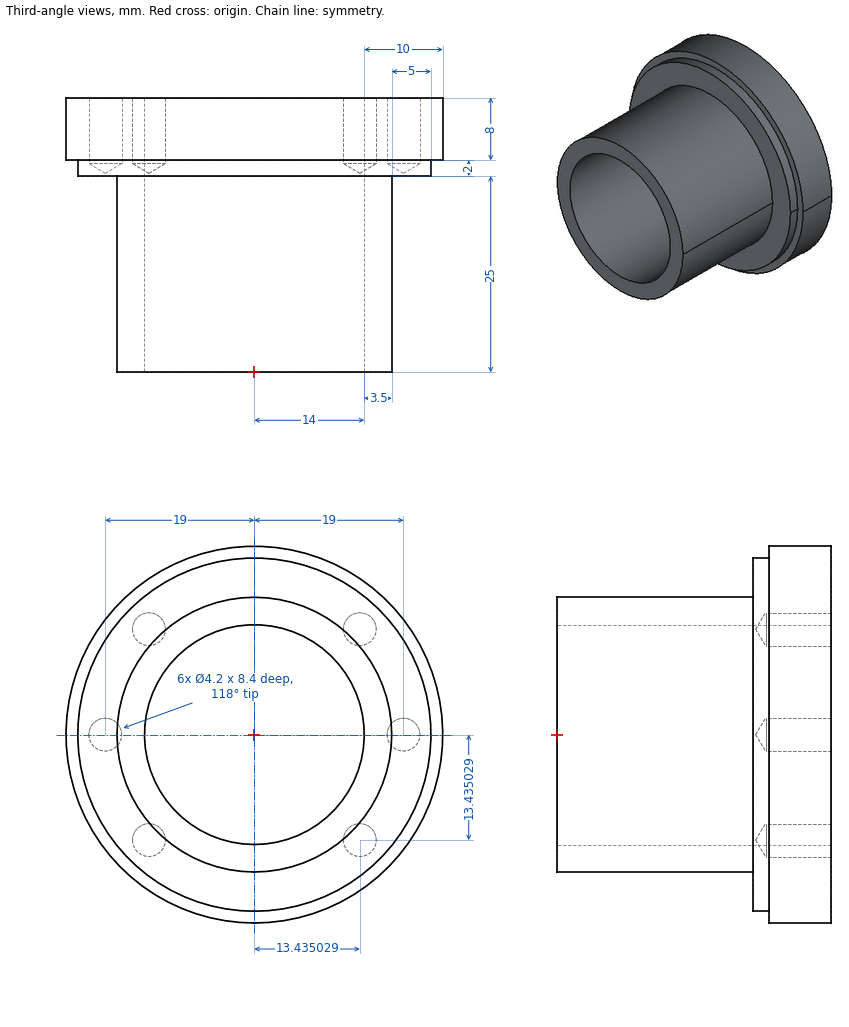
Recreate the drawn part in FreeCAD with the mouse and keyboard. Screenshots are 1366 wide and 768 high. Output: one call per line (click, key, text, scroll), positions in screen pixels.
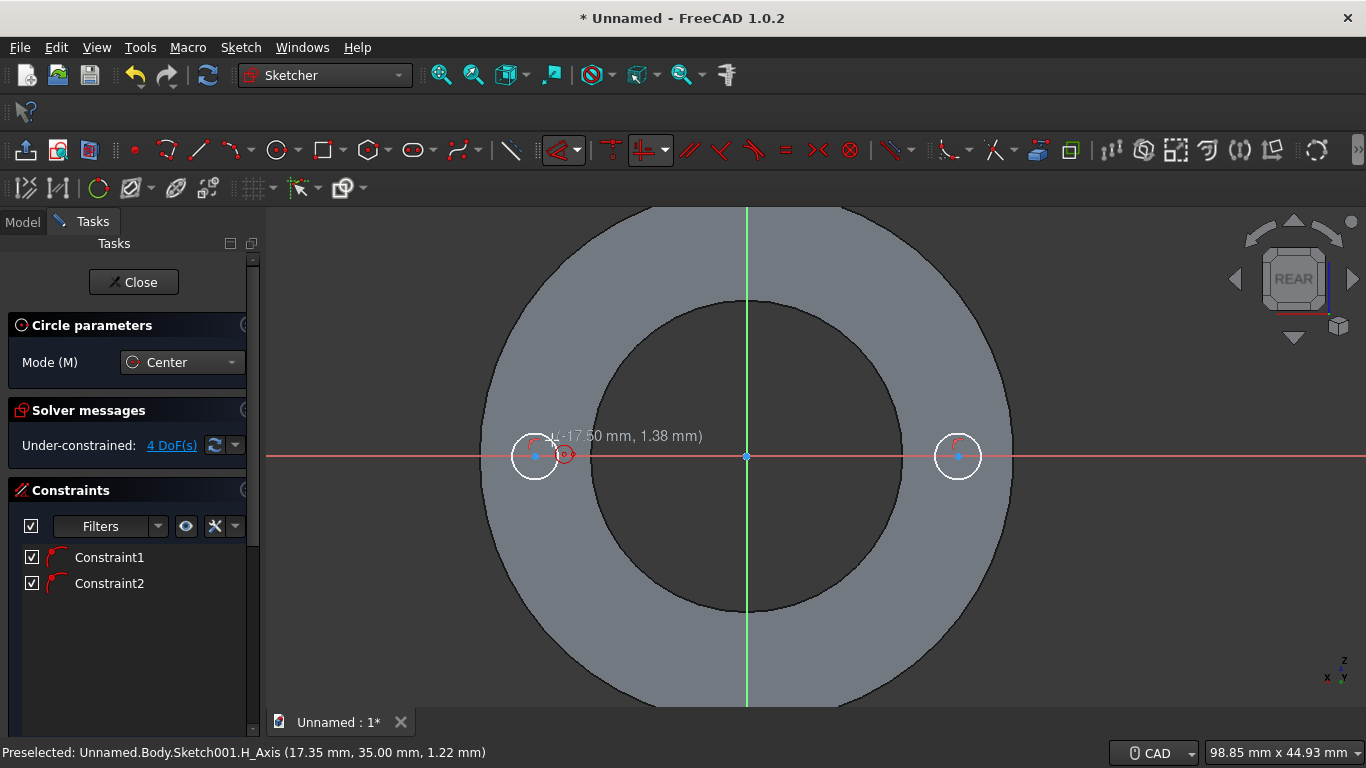
click(597, 606)
click(614, 589)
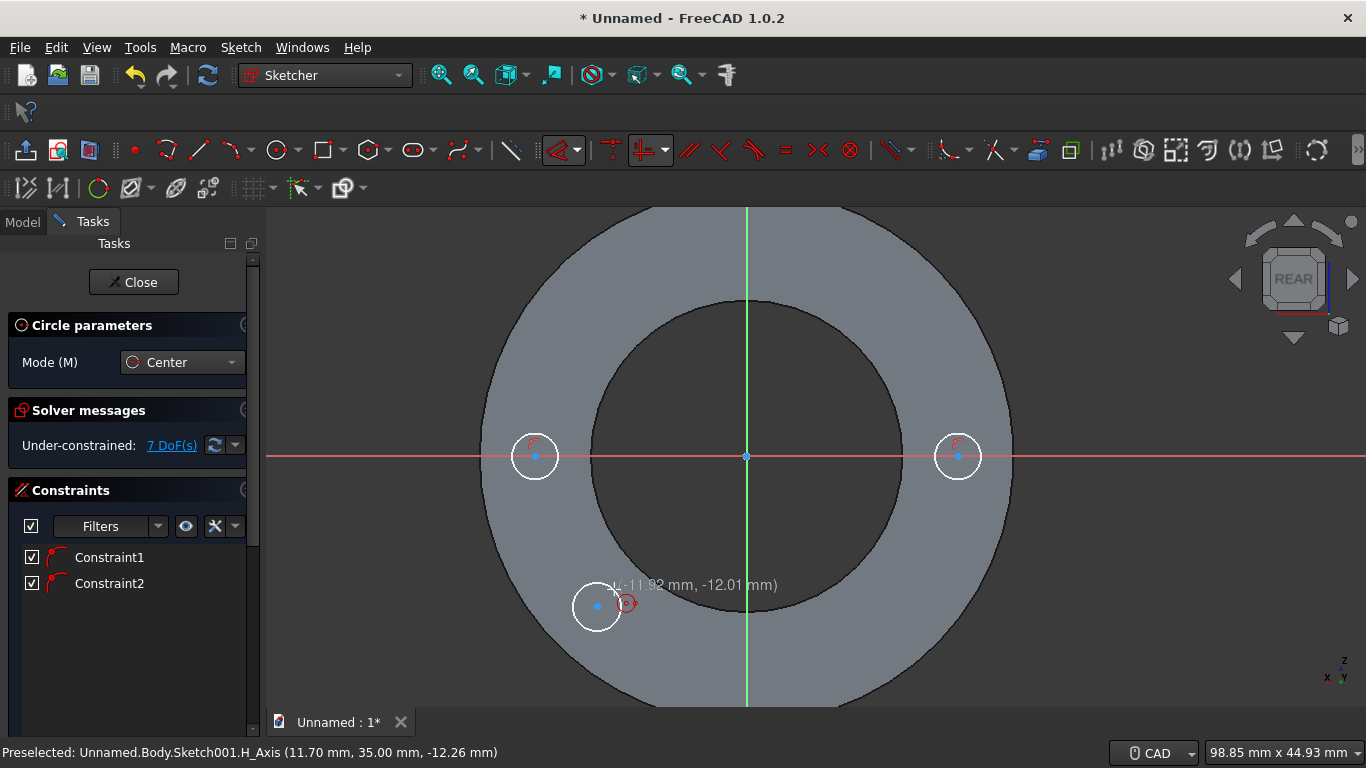
click(597, 307)
click(614, 290)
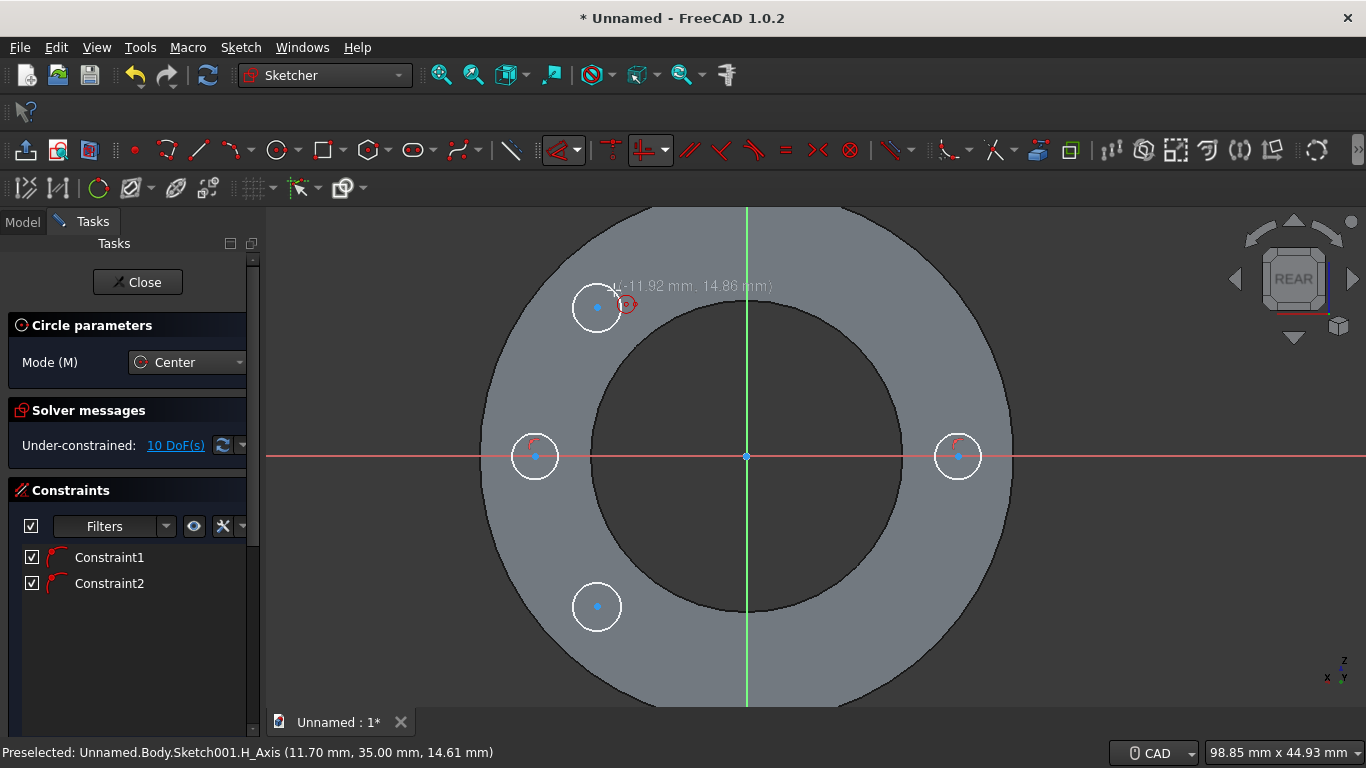
click(896, 307)
click(913, 290)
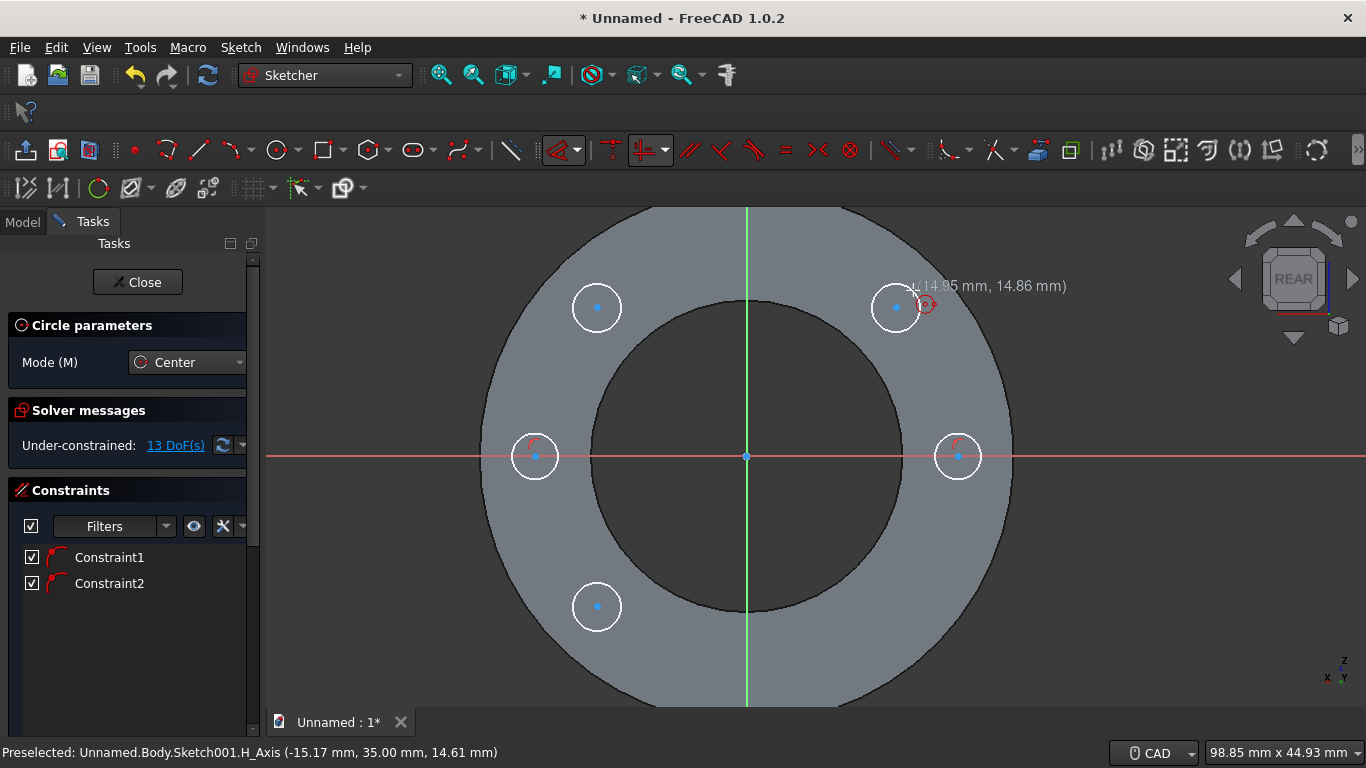
click(896, 606)
click(913, 589)
key(Escape)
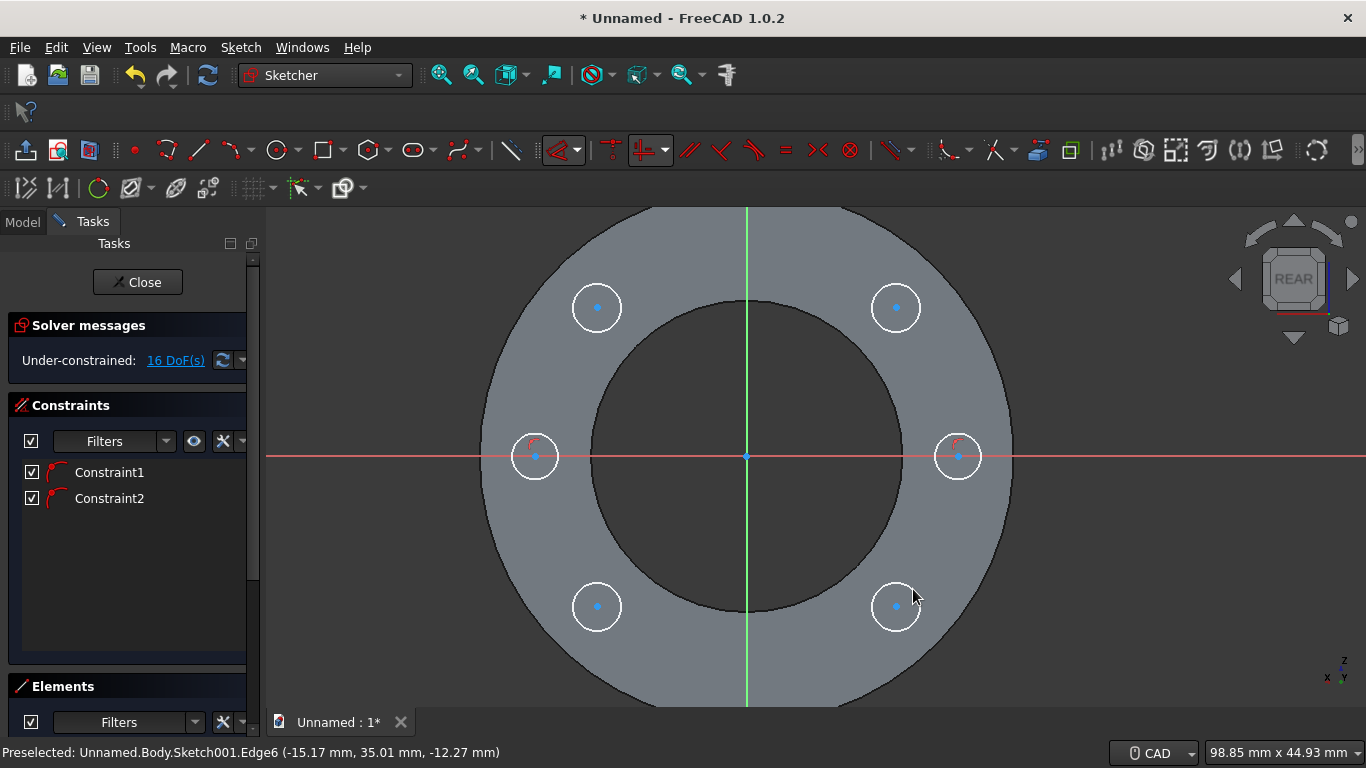
click(974, 440)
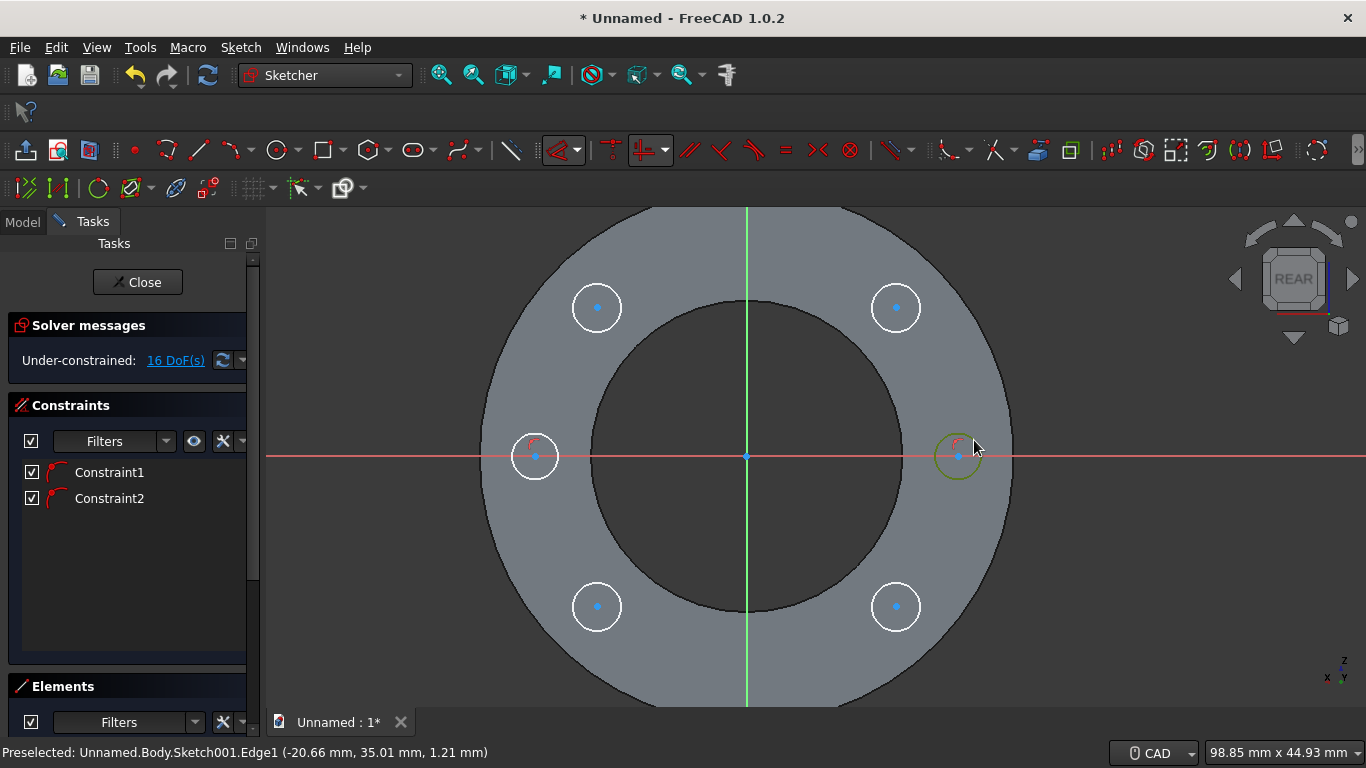
click(551, 440)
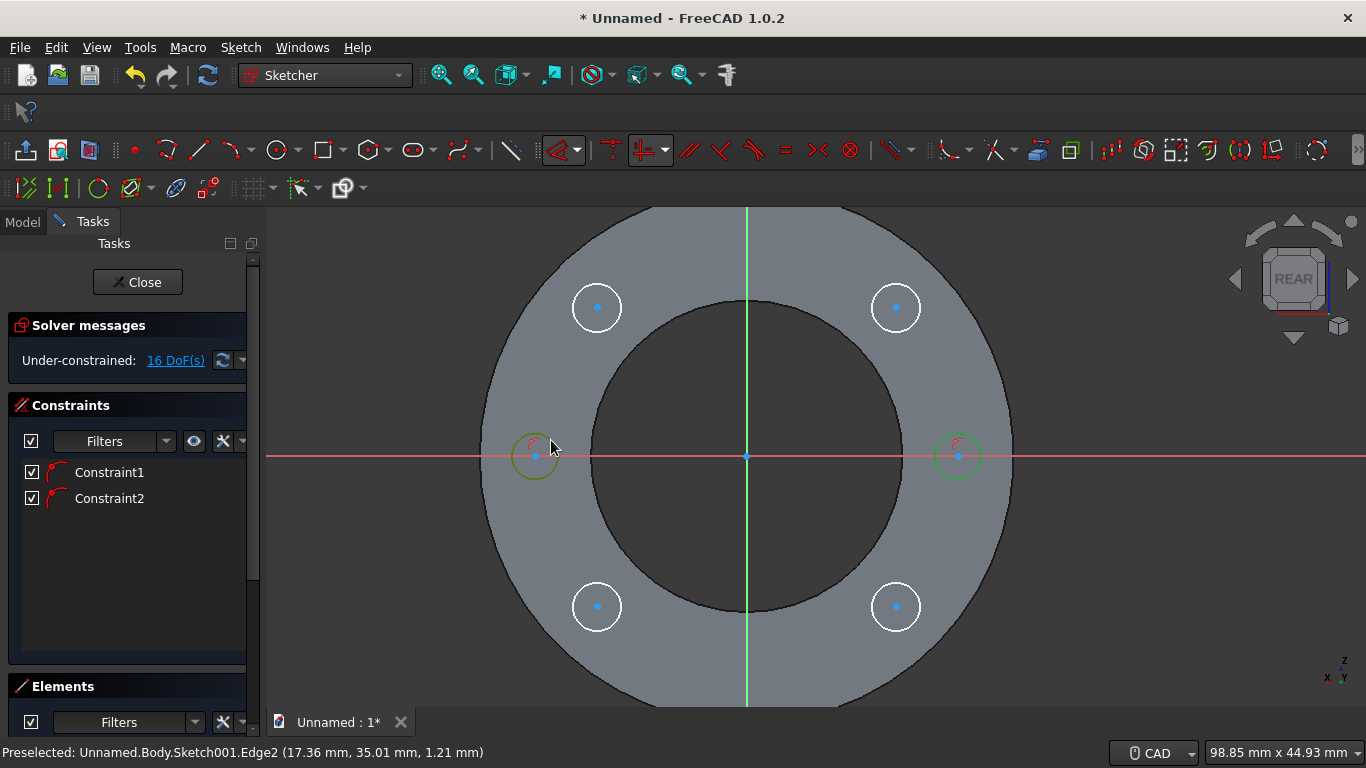
click(614, 590)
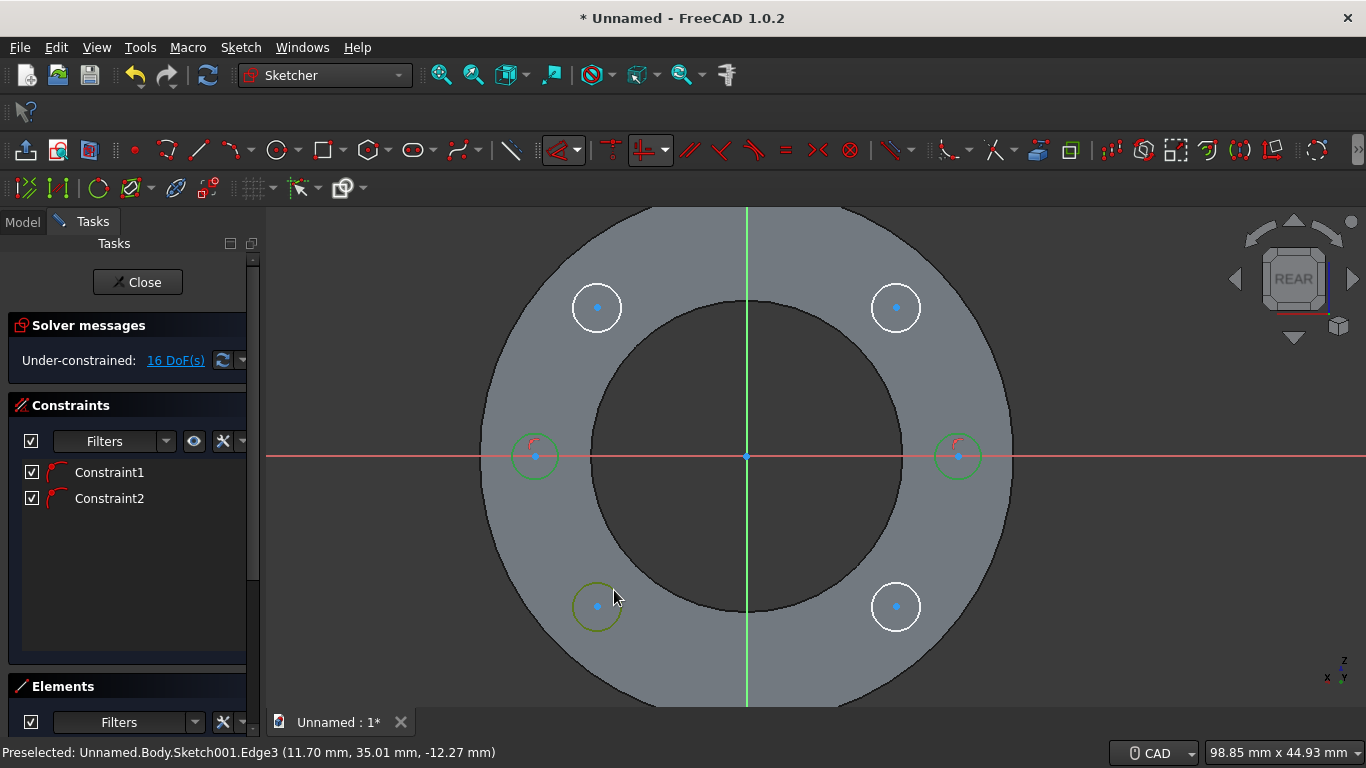
click(614, 291)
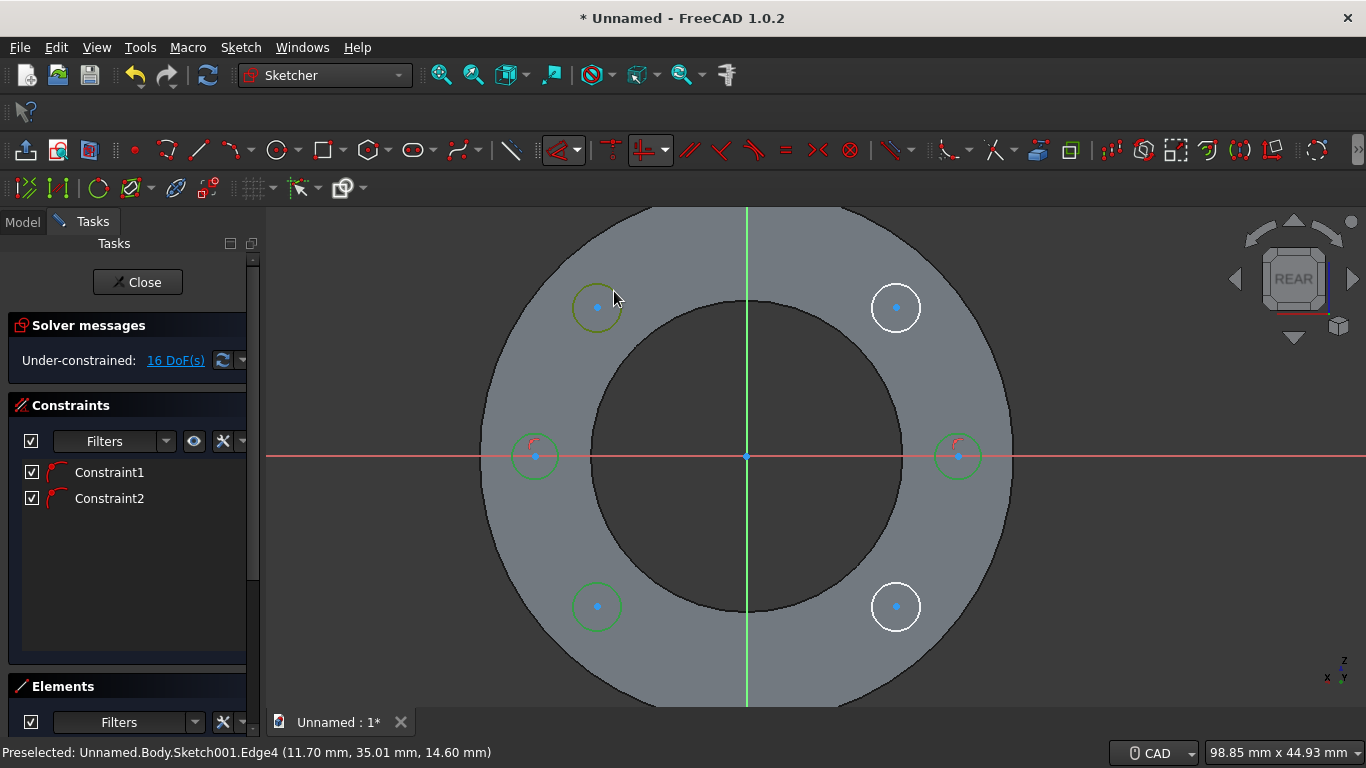
click(913, 291)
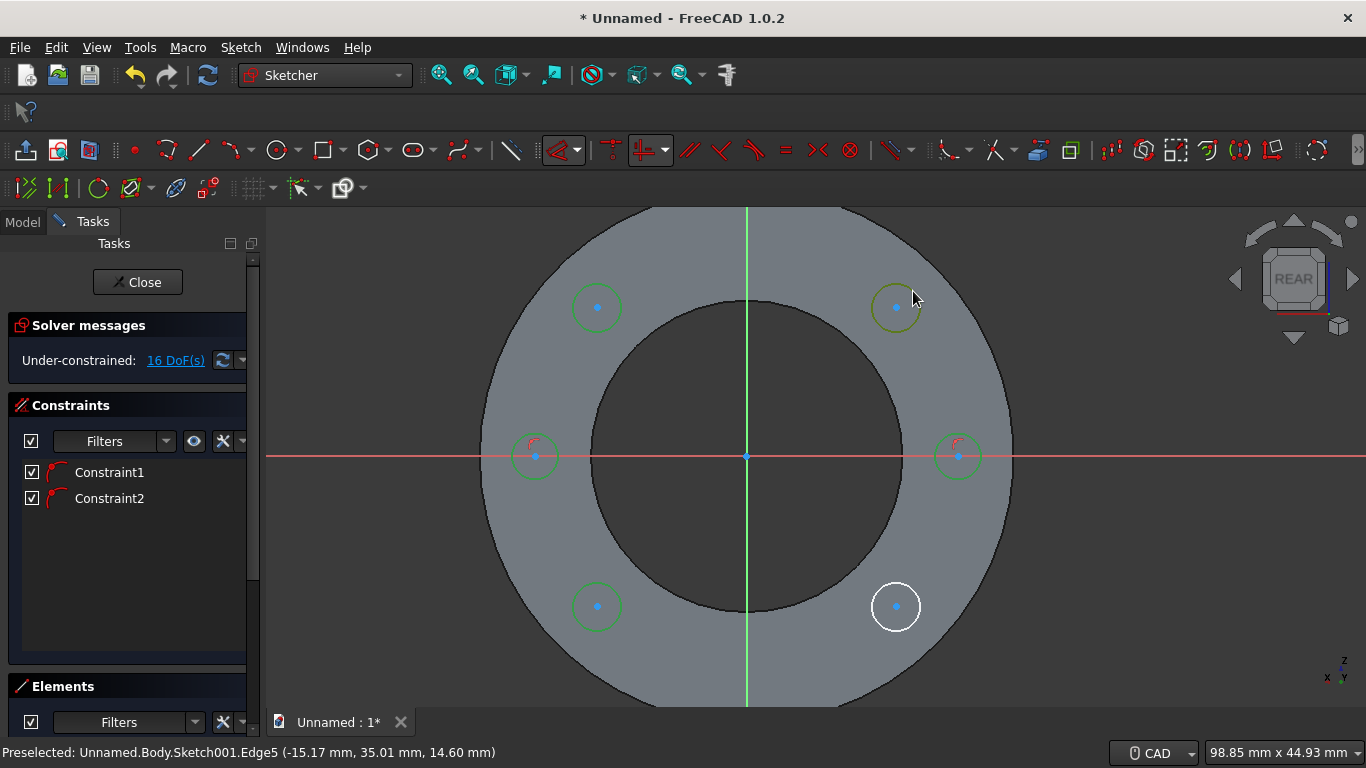
click(913, 590)